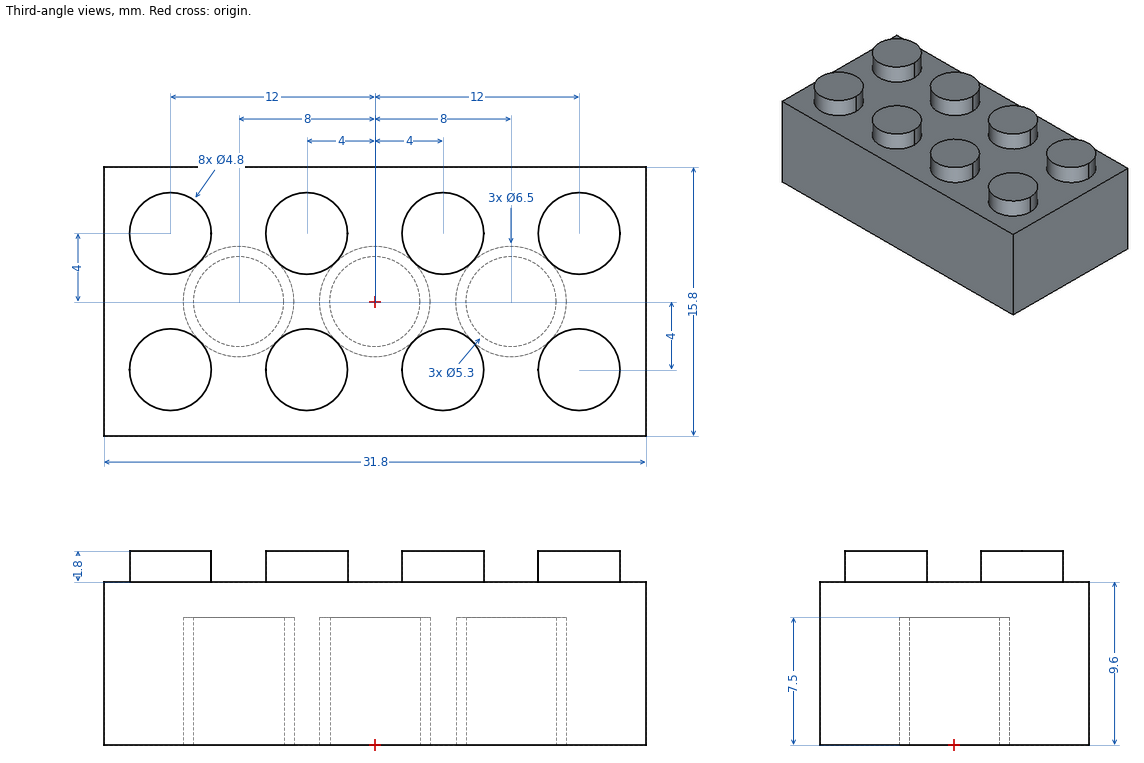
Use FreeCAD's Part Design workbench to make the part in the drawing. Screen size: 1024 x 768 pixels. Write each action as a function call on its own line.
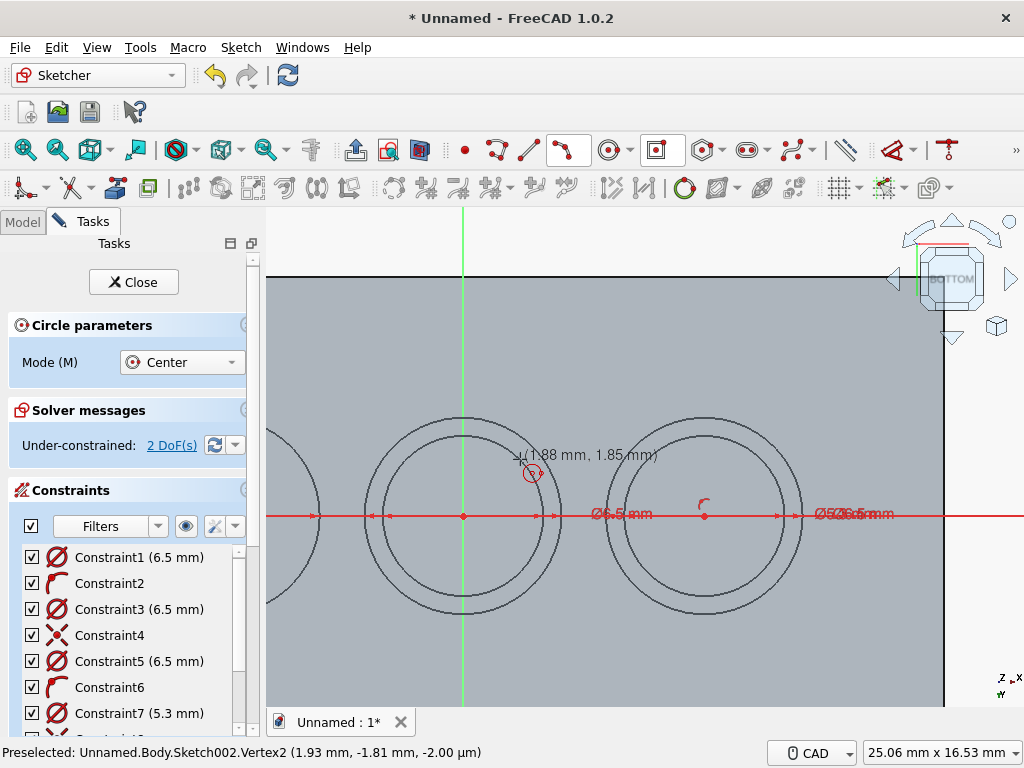
scroll(715, 385, down, 3)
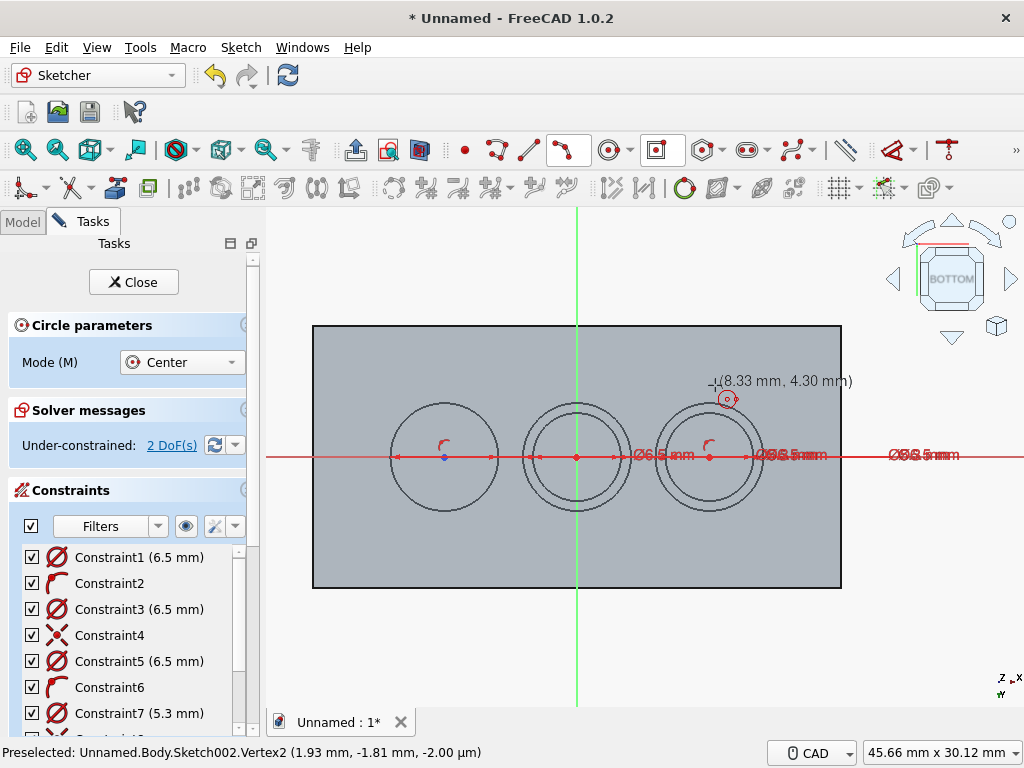
click(444, 457)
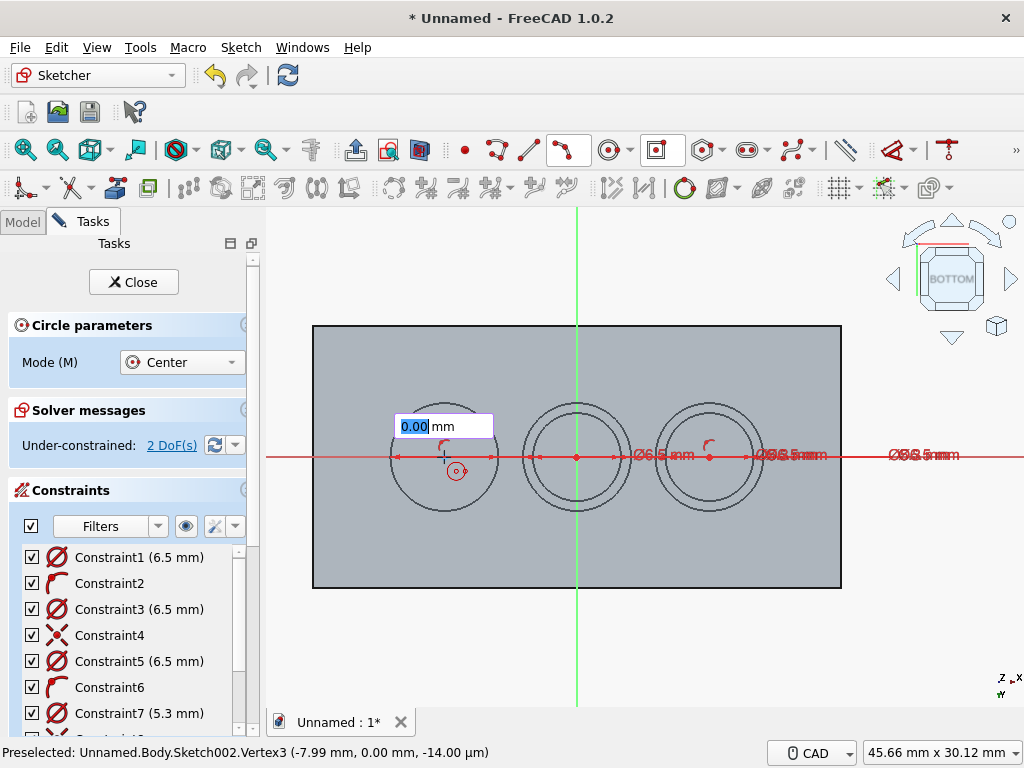
scroll(459, 416, up, 3)
move(459, 415)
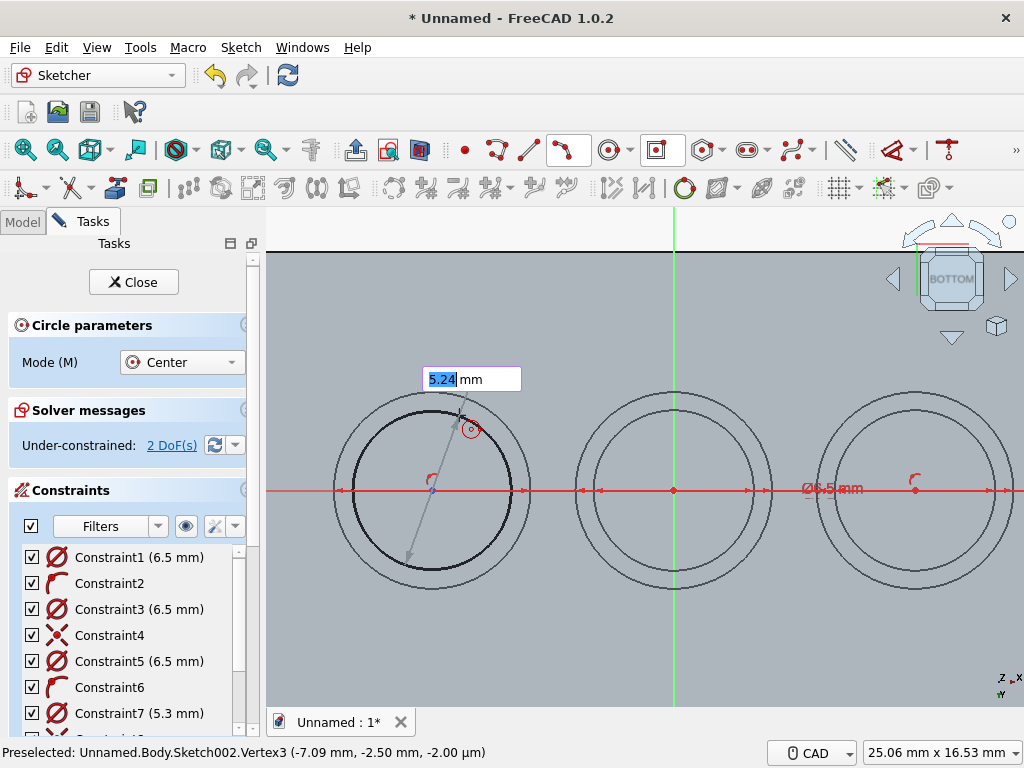
text(5.3)
key(Return)
key(Escape)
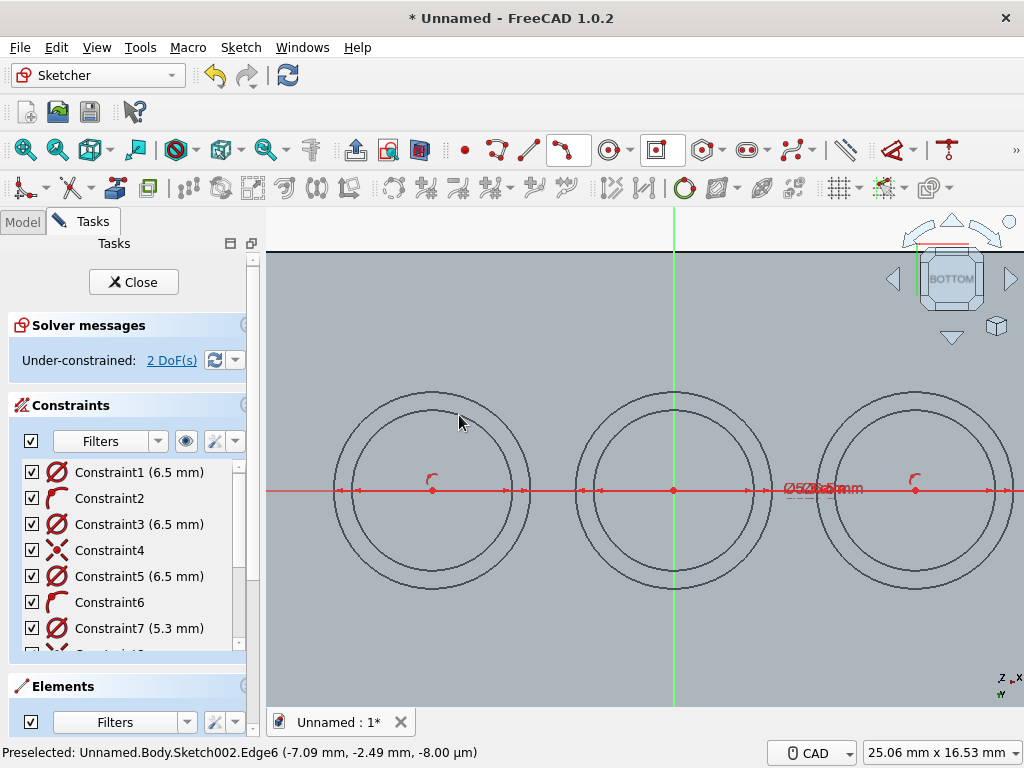
click(892, 150)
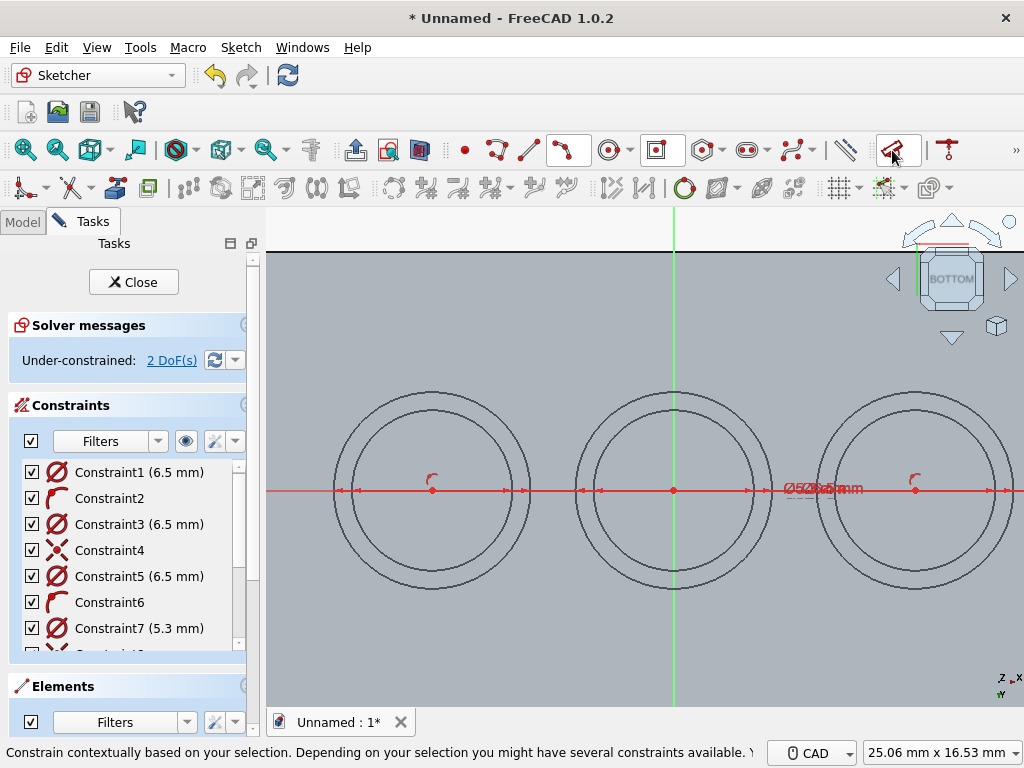
scroll(458, 416, down, 3)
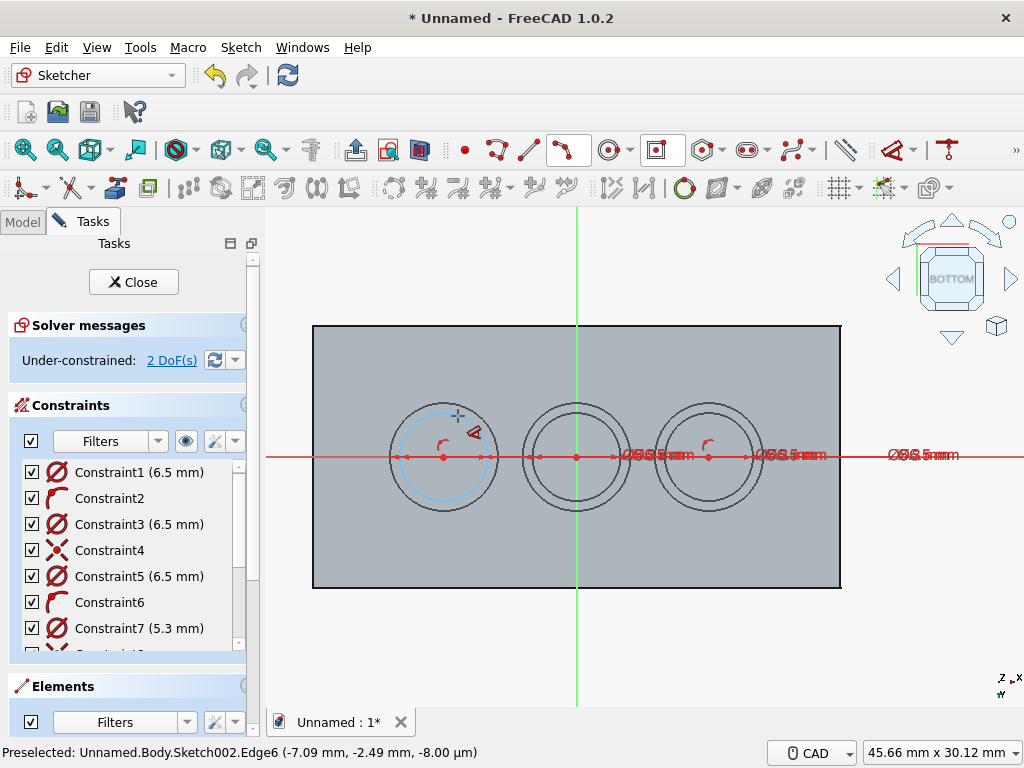
click(709, 457)
click(643, 491)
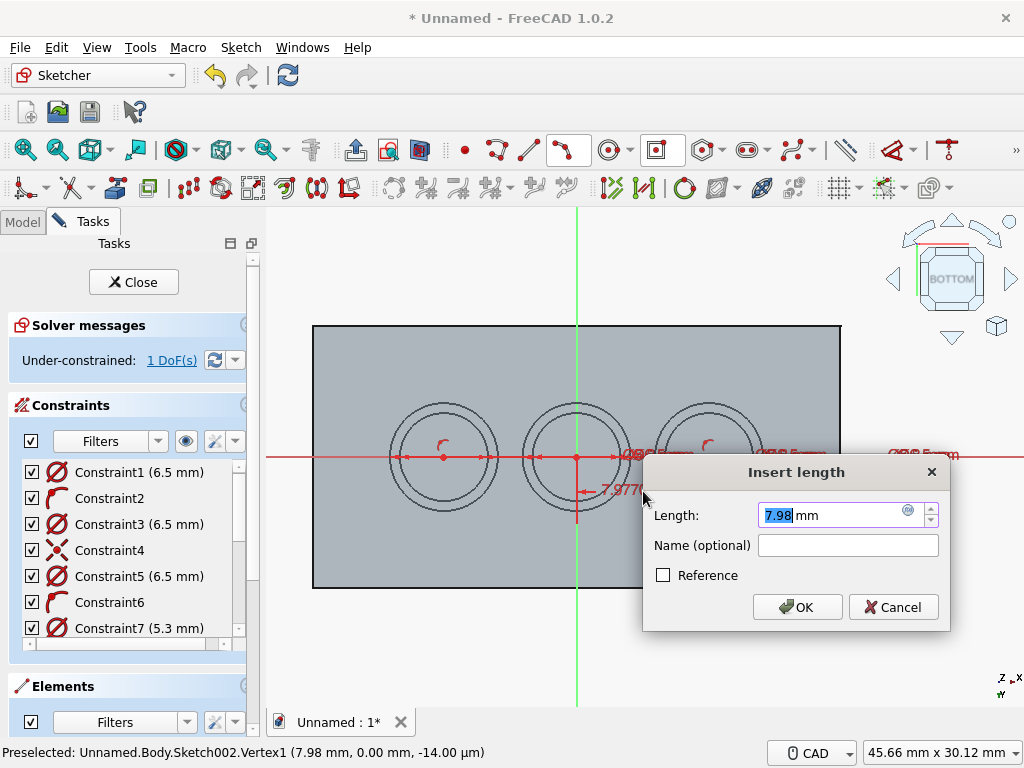
text(8)
key(Return)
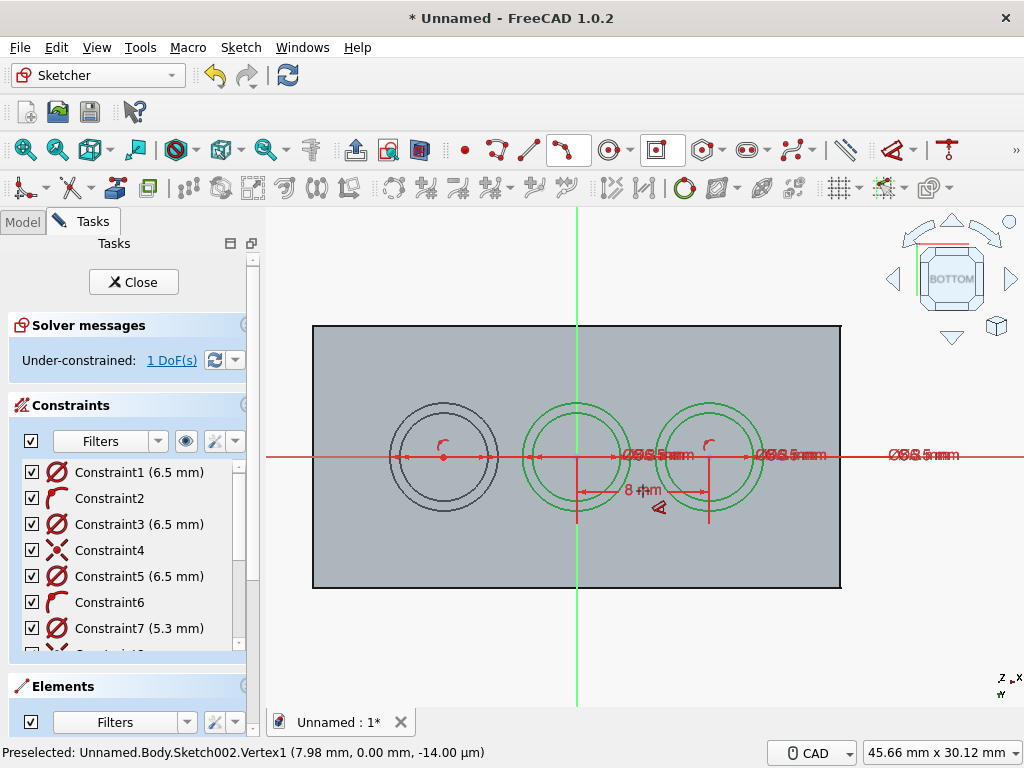
click(444, 457)
click(510, 491)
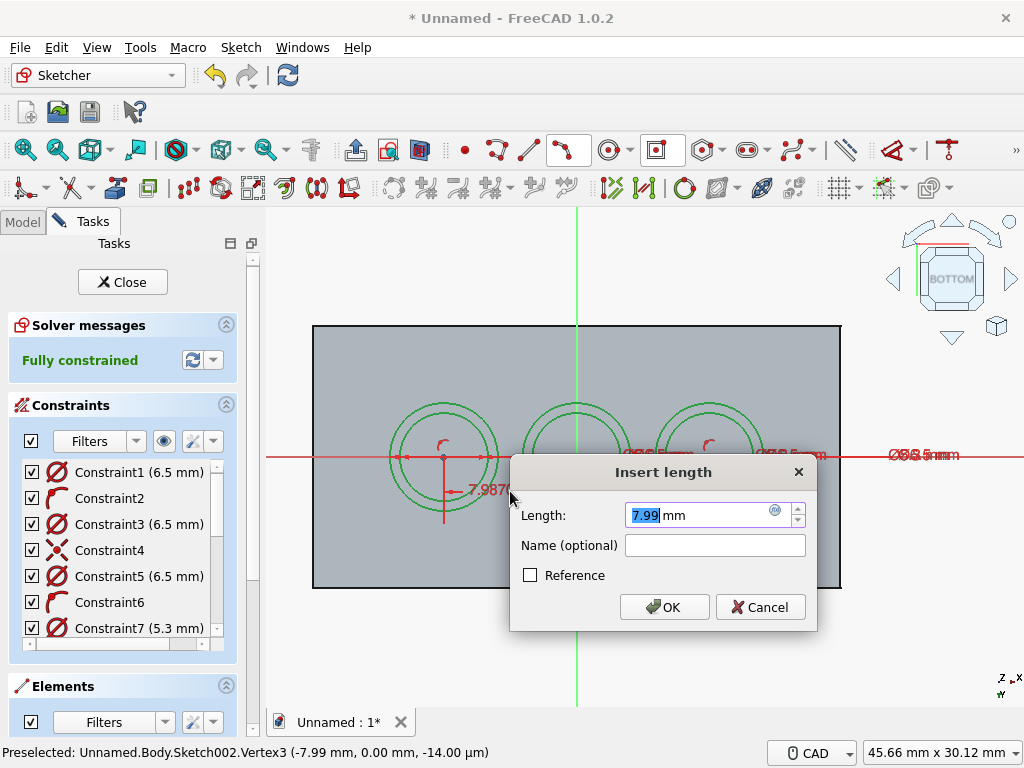
text(8)
key(Return)
key(Escape)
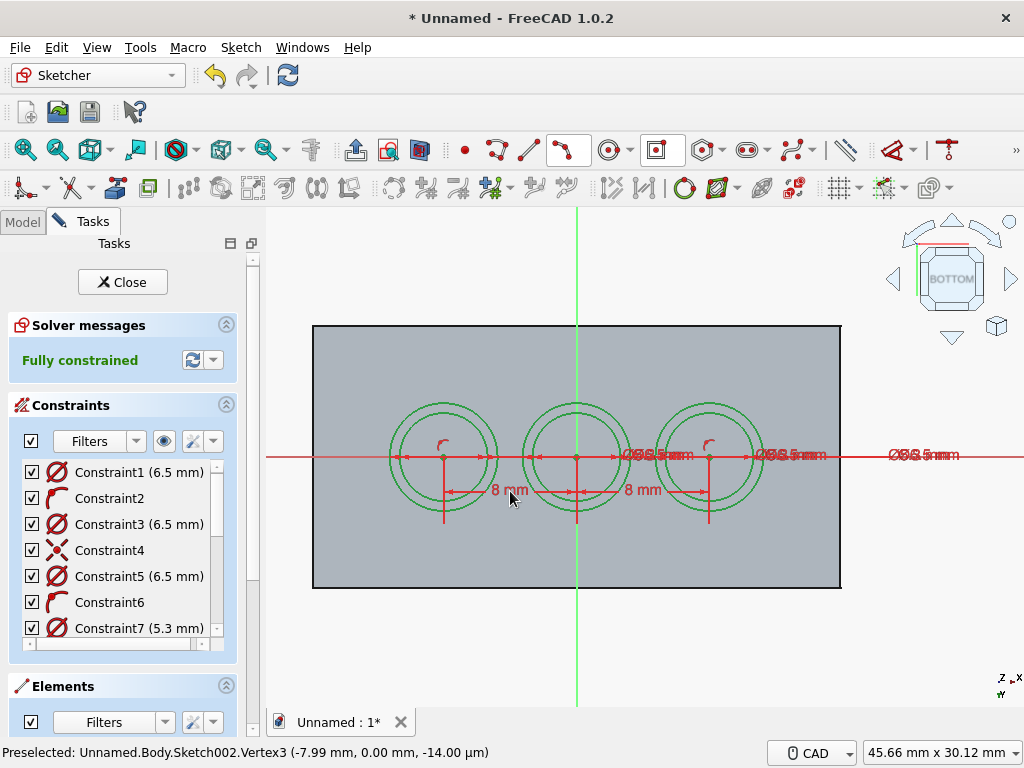
click(123, 282)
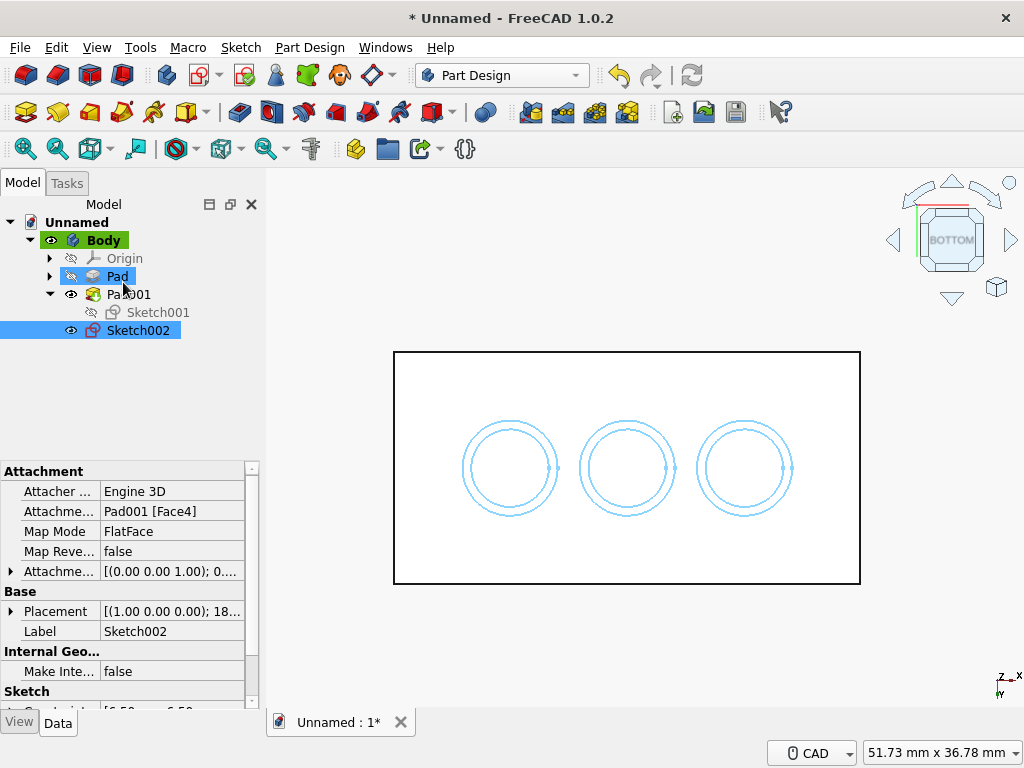
click(240, 112)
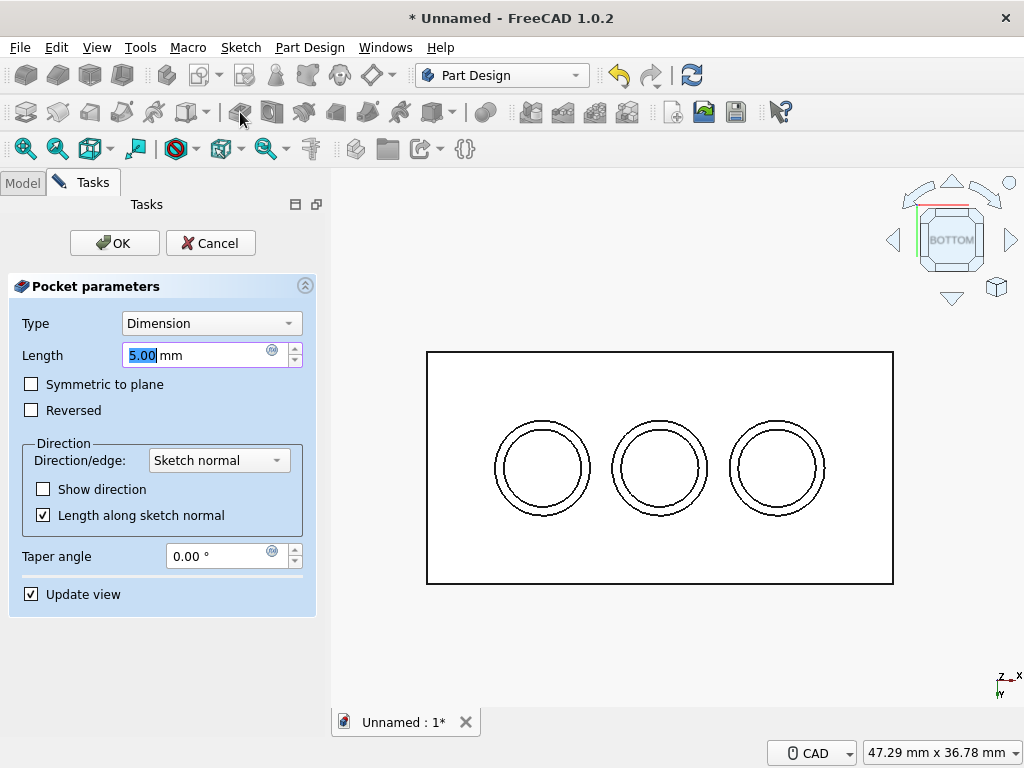
click(212, 324)